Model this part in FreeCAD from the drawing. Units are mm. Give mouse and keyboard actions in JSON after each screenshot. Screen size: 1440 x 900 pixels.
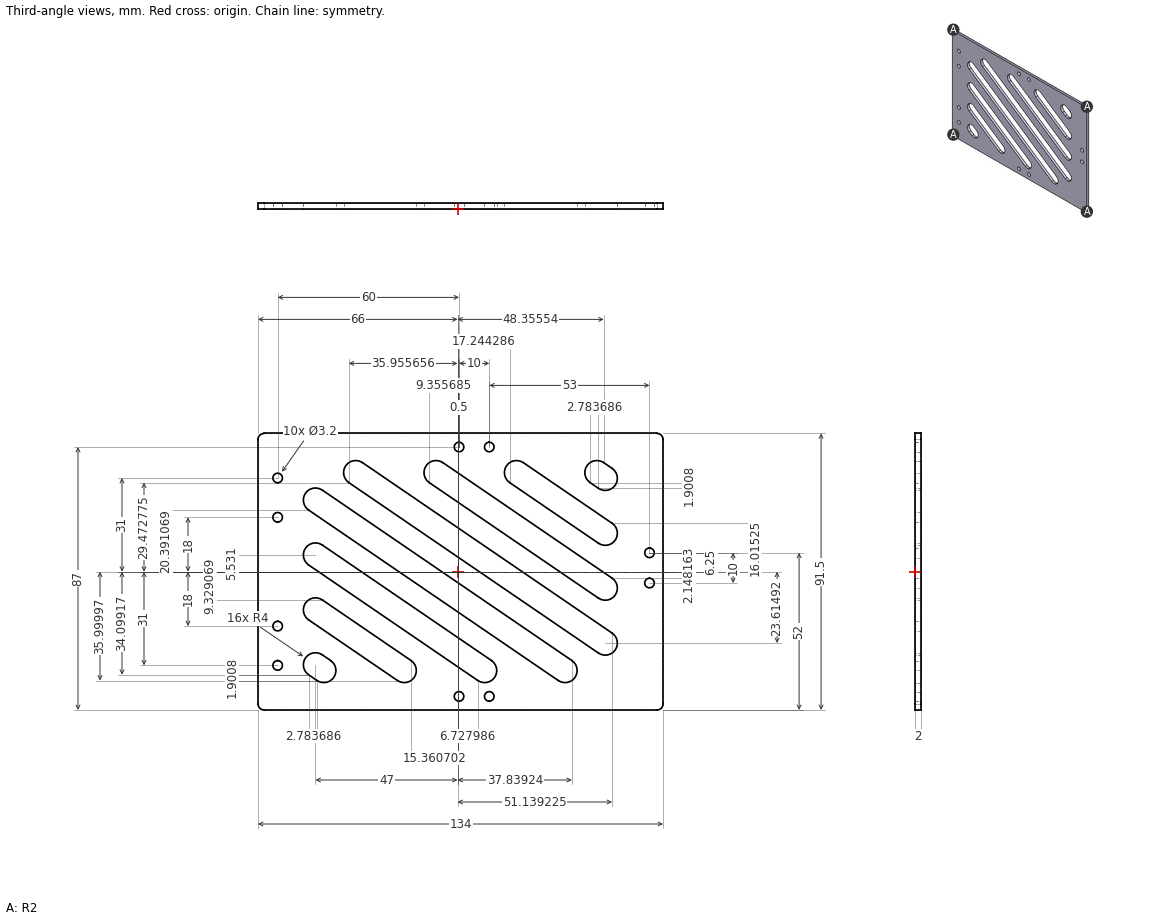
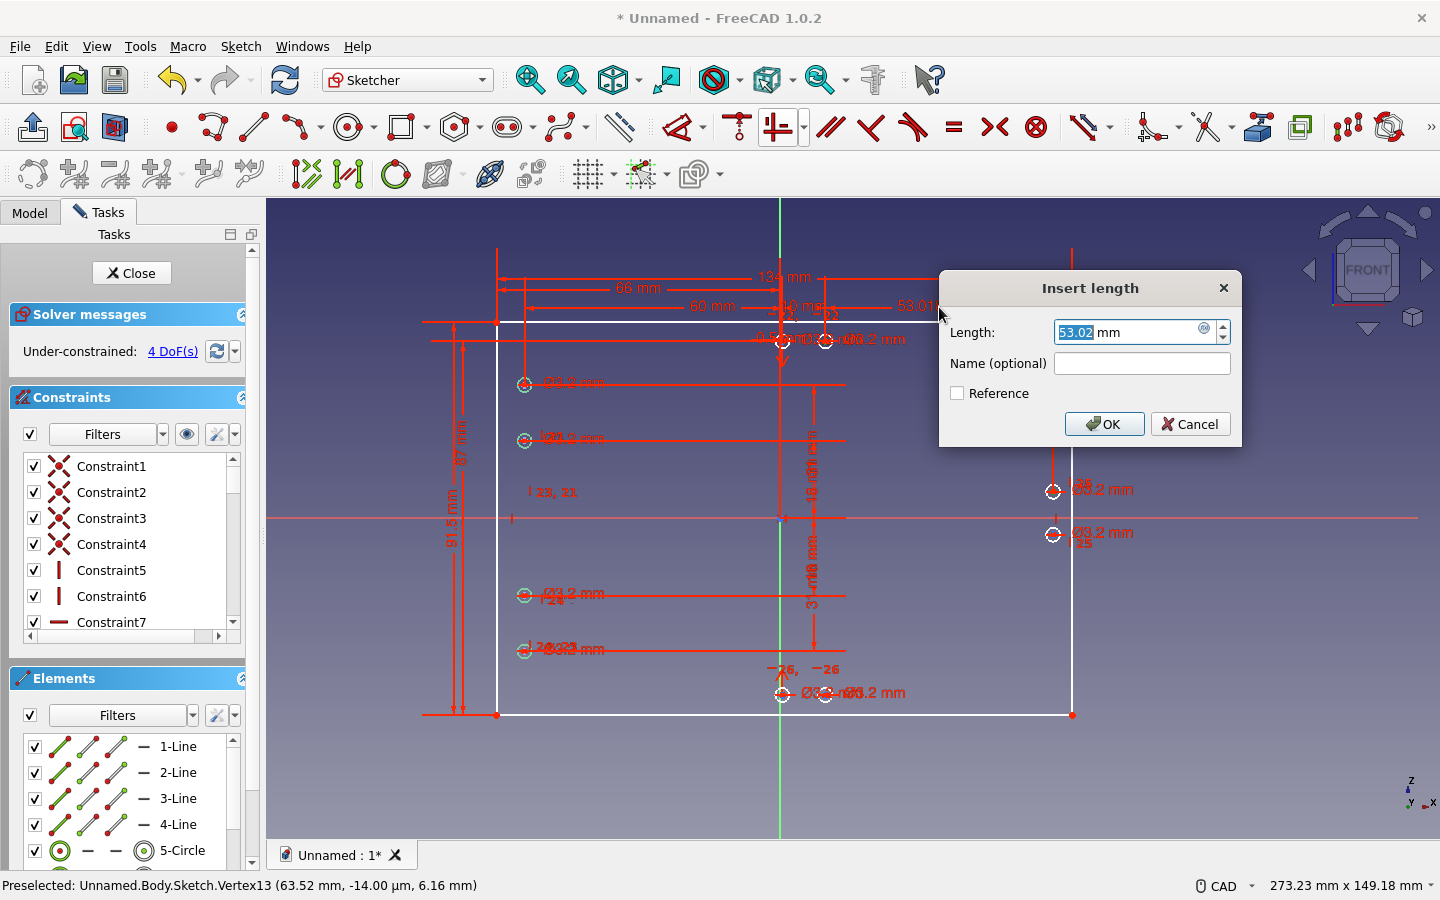
{"action": "type", "text": "53"}
{"action": "key", "text": "Return"}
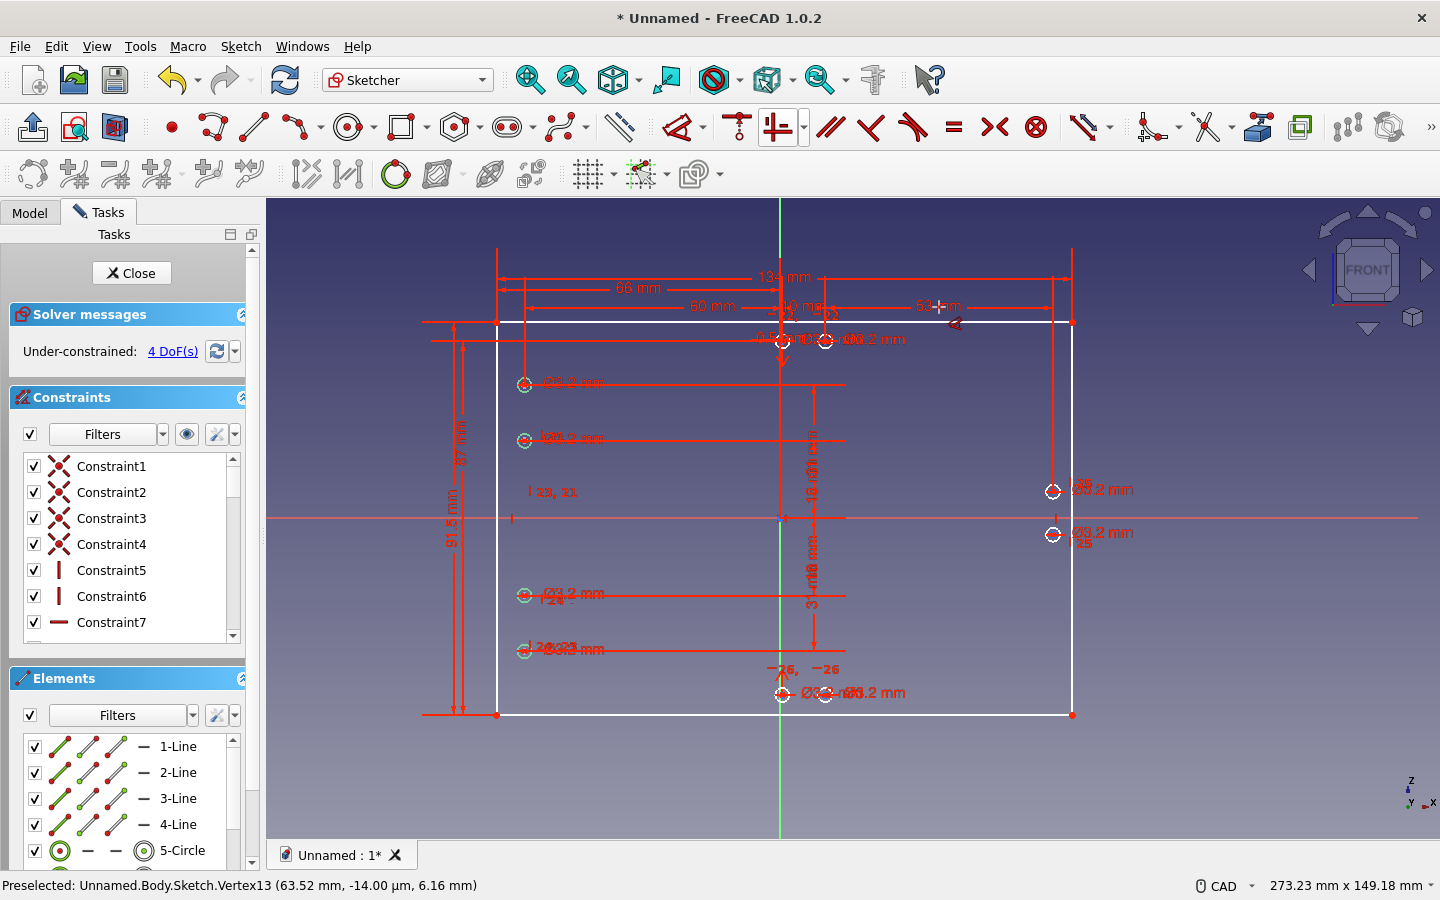
{"action": "left_click", "coordinate": [1072, 715]}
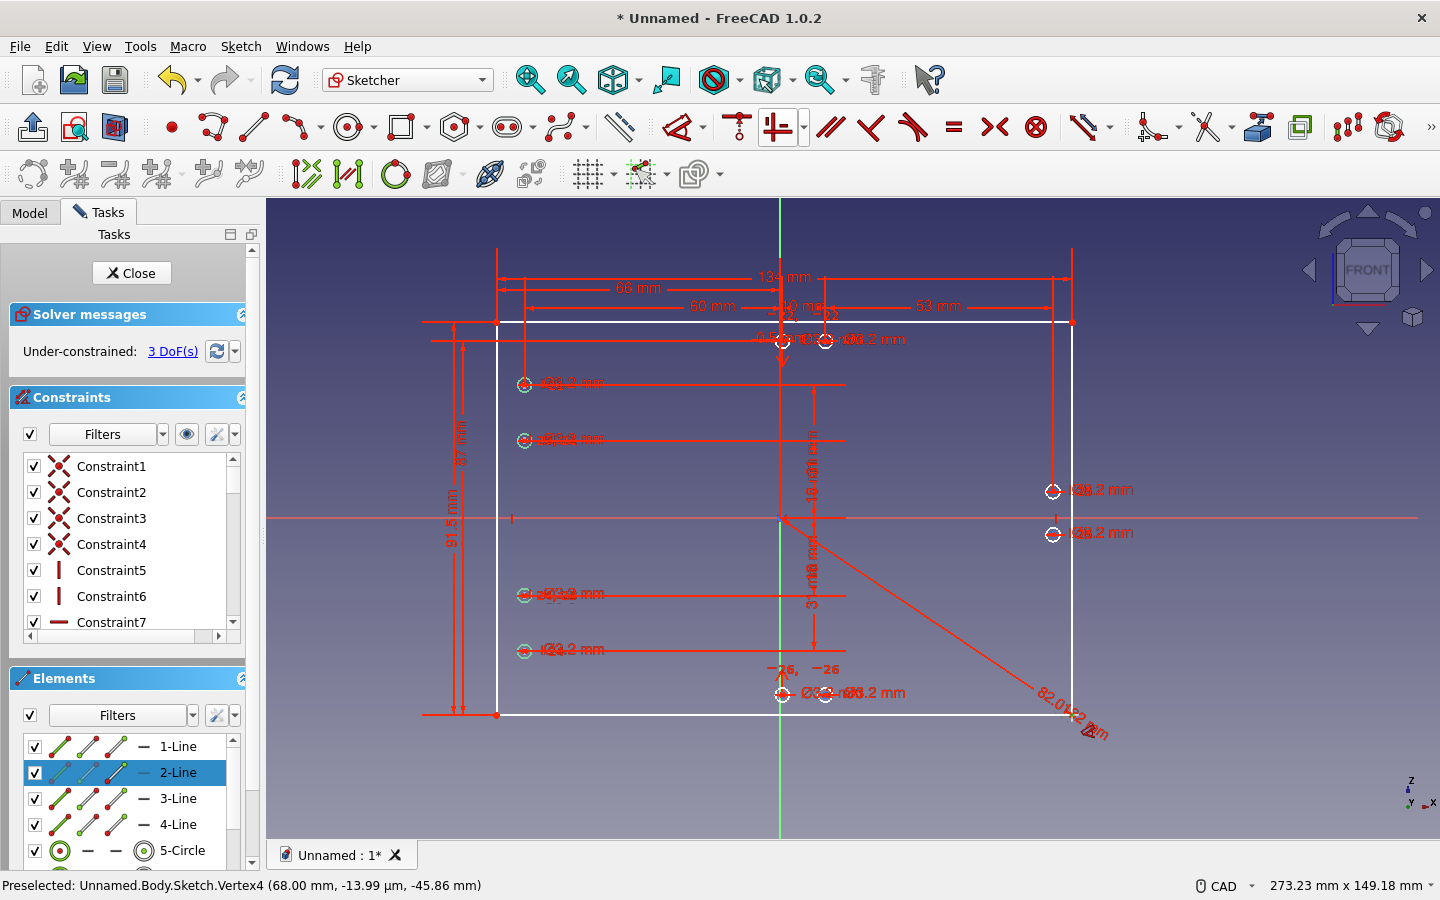
{"action": "left_click", "coordinate": [1053, 492]}
{"action": "left_click", "coordinate": [1106, 604]}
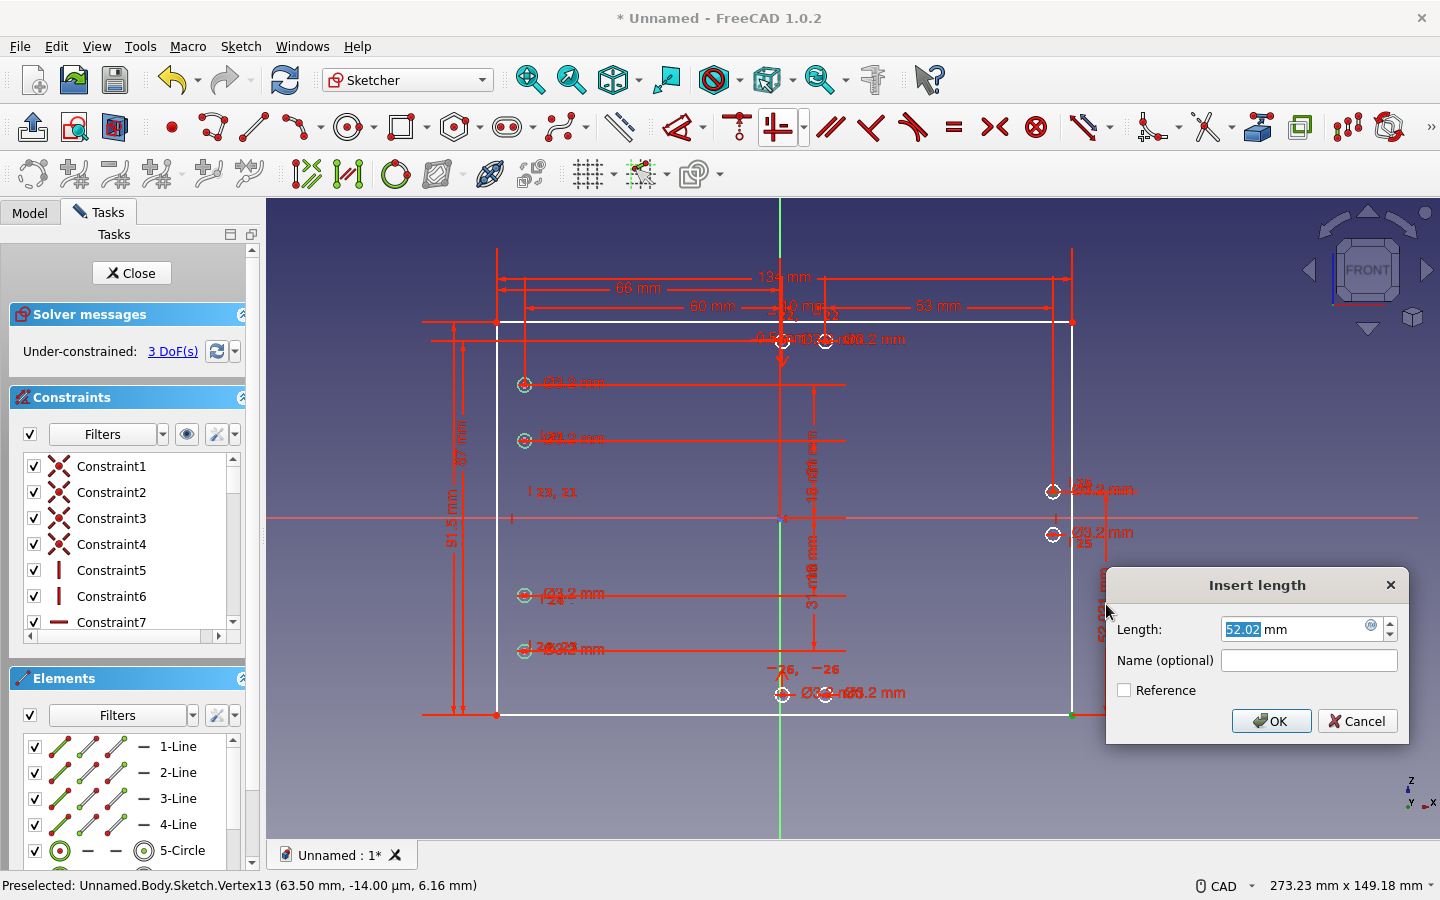
{"action": "type", "text": "52"}
{"action": "key", "text": "Return"}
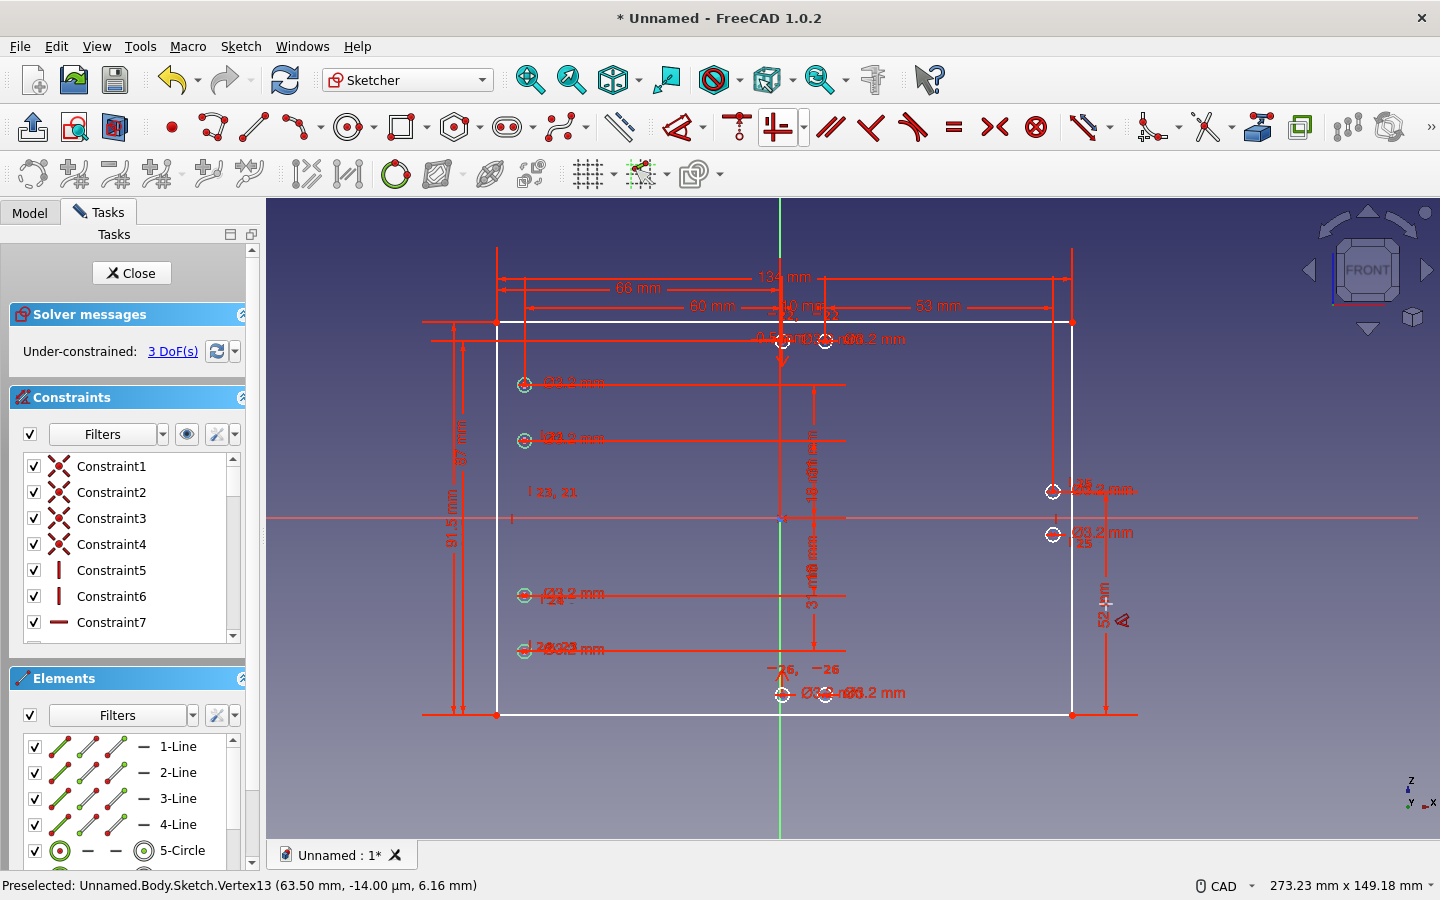
{"action": "left_click", "coordinate": [1053, 492]}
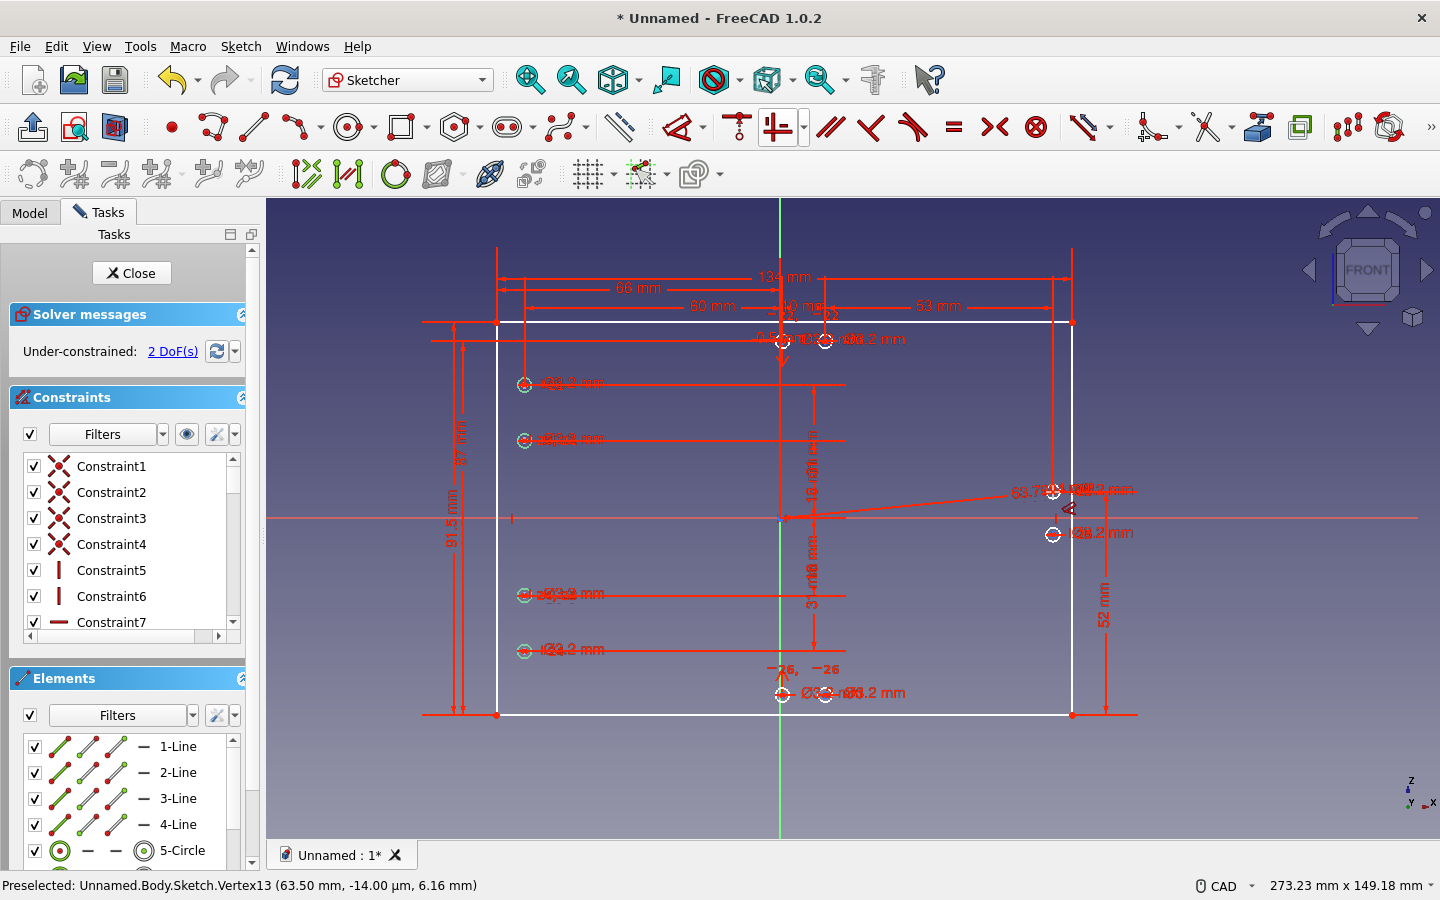
{"action": "left_click", "coordinate": [1053, 535]}
{"action": "left_click", "coordinate": [1087, 503]}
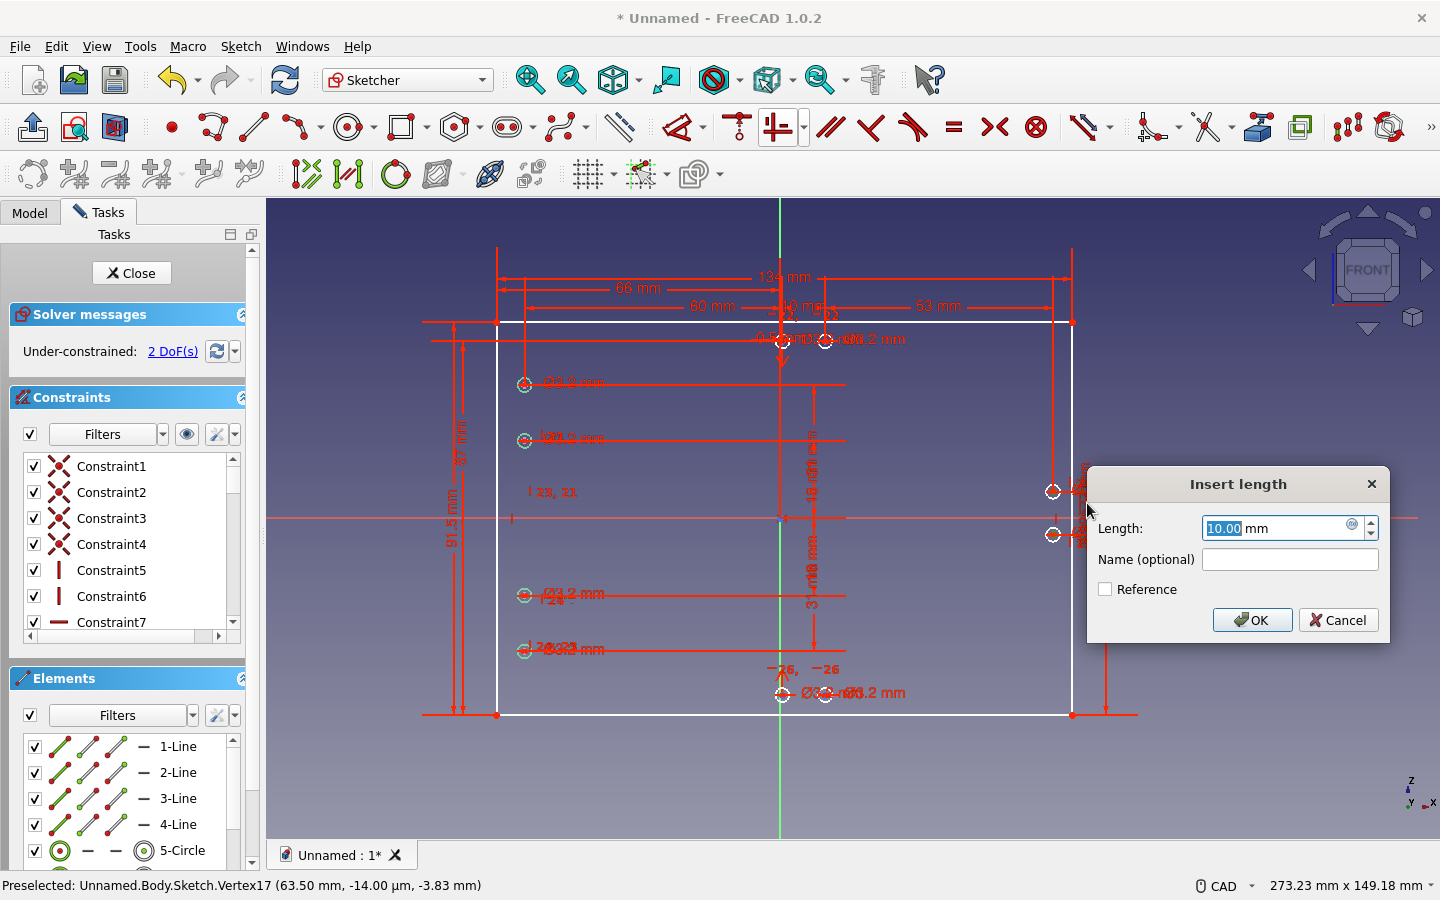
{"action": "type", "text": "10"}
{"action": "key", "text": "Return"}